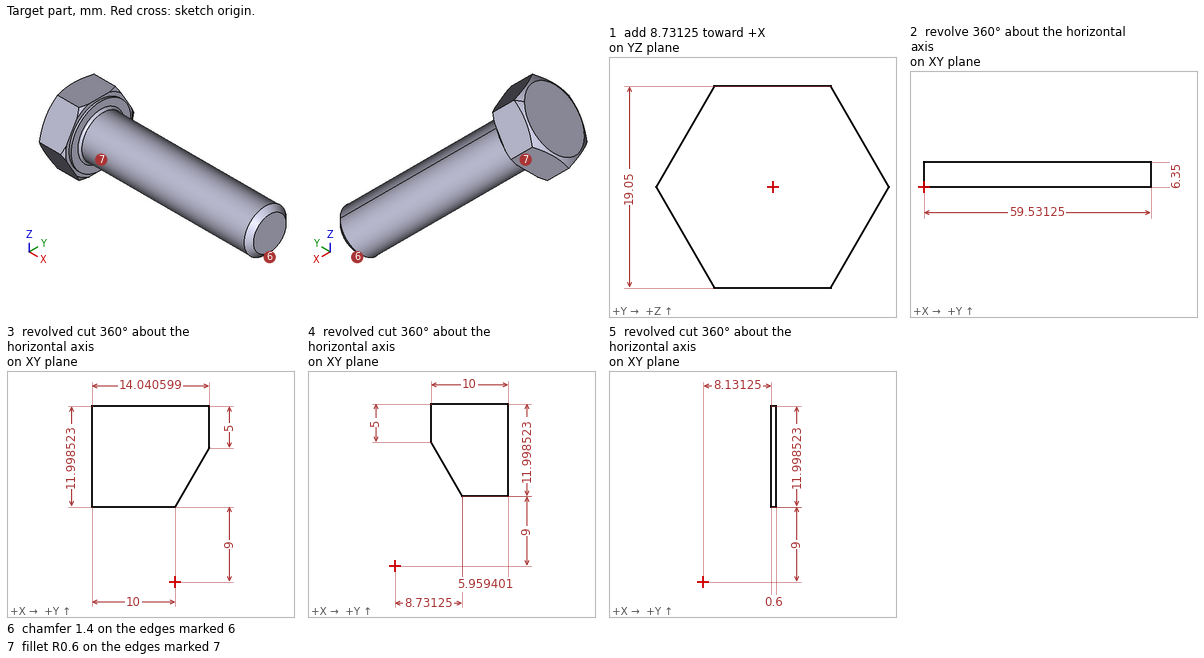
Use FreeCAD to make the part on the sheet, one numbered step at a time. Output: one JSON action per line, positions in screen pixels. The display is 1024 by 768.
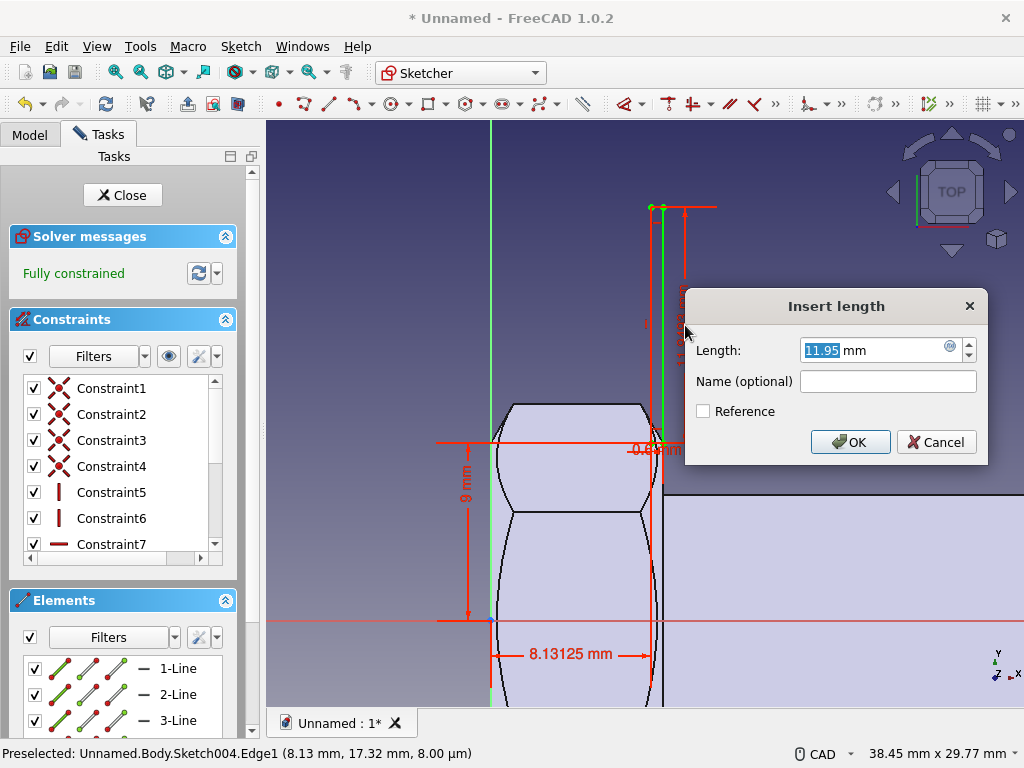
{"action": "type", "text": "11.998523"}
{"action": "key", "text": "Return"}
{"action": "key", "text": "Escape"}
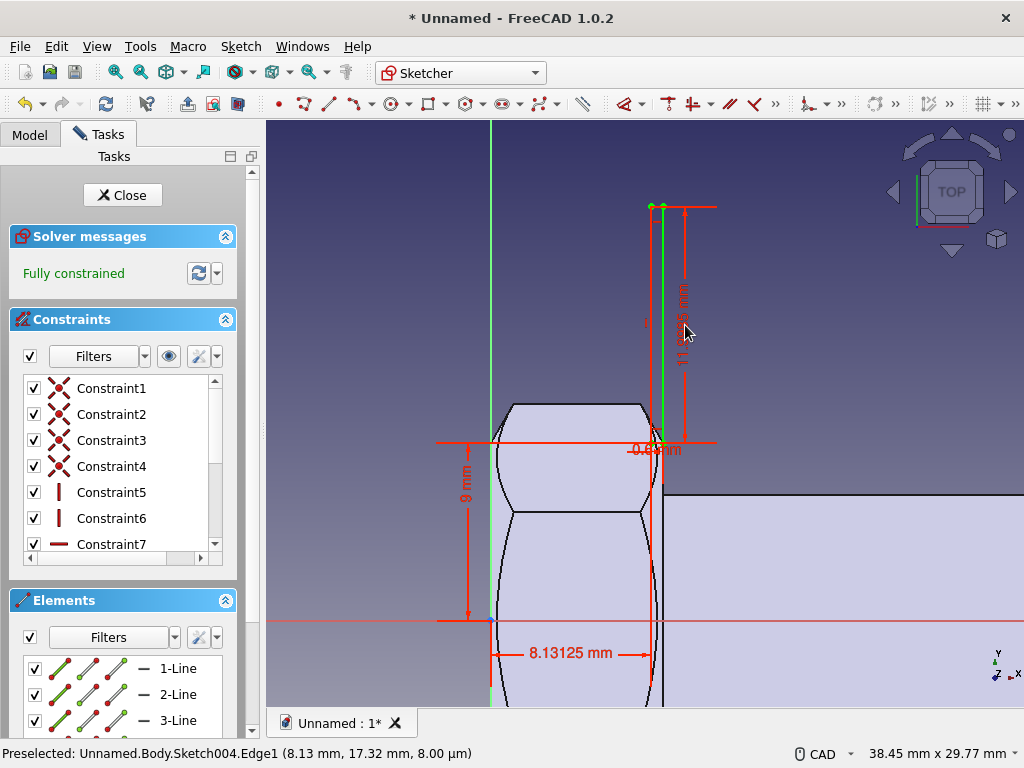
{"action": "left_click", "coordinate": [123, 195]}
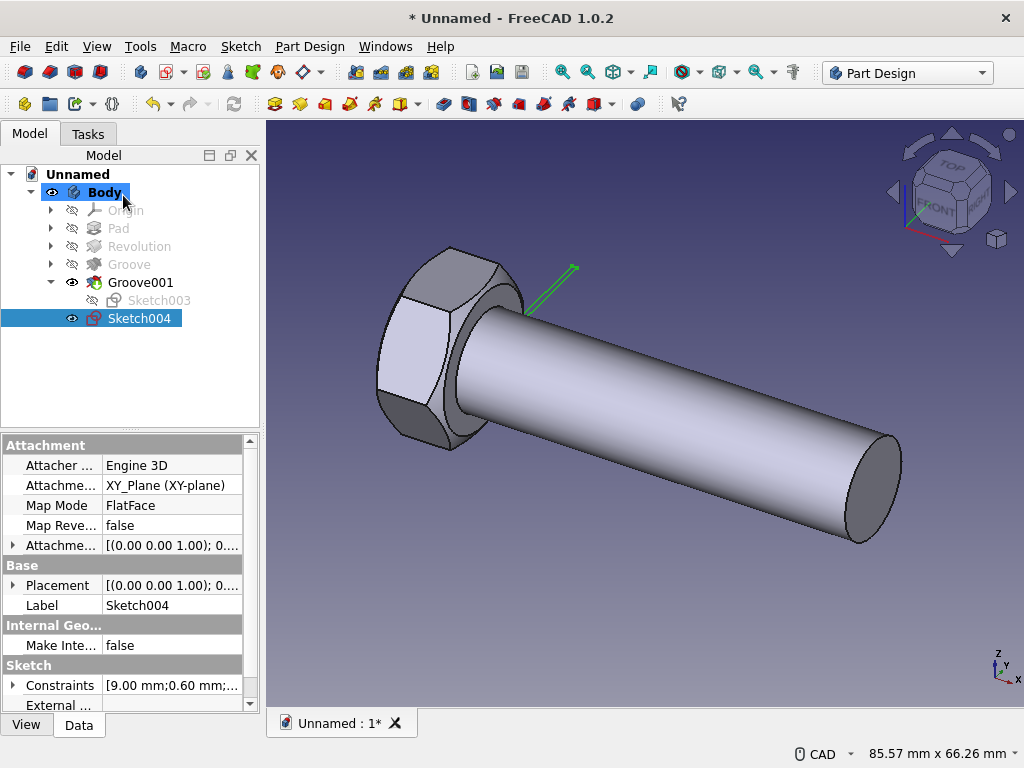
{"action": "left_click", "coordinate": [494, 104]}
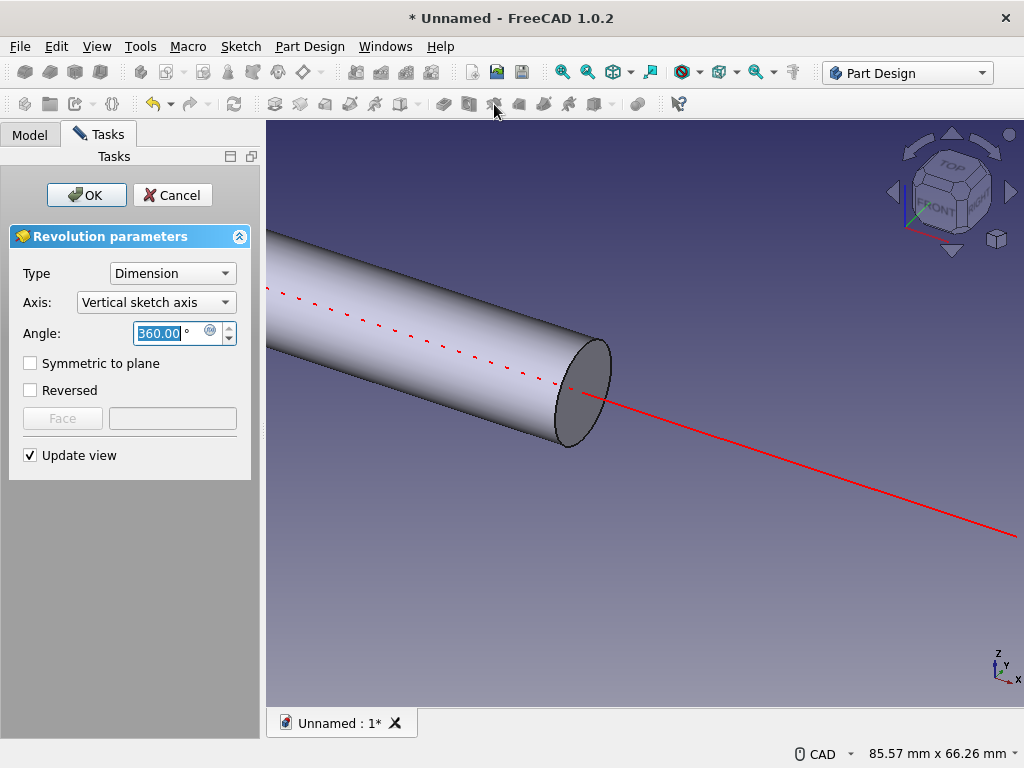
{"action": "left_click", "coordinate": [157, 302]}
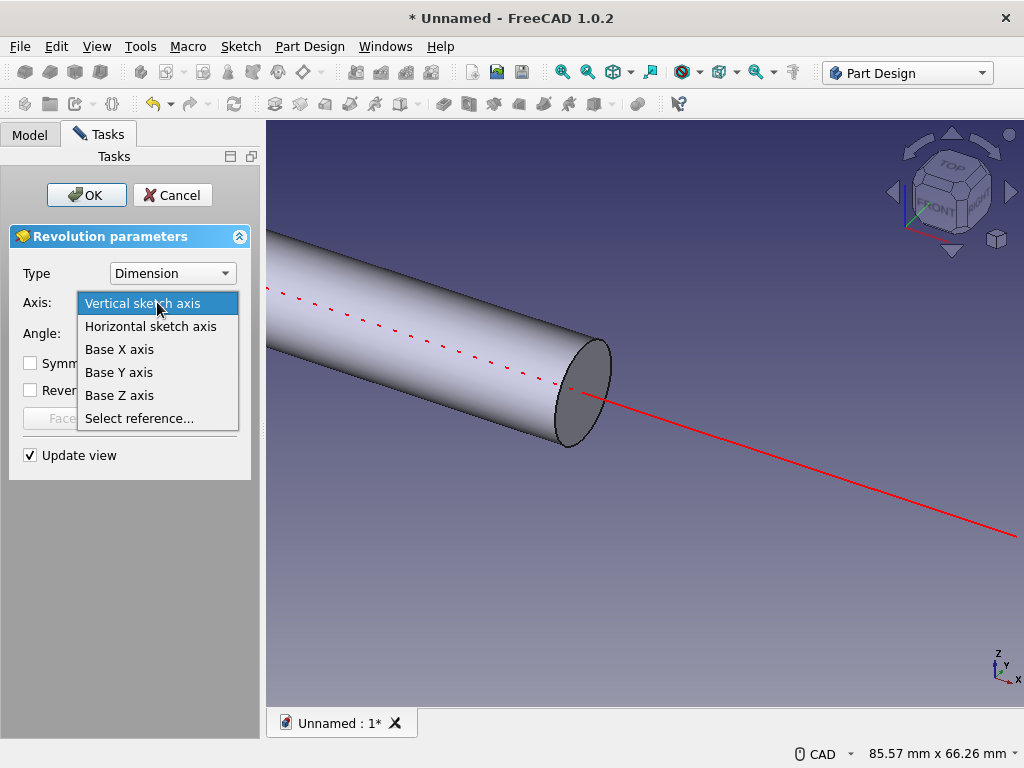
{"action": "left_click", "coordinate": [156, 326]}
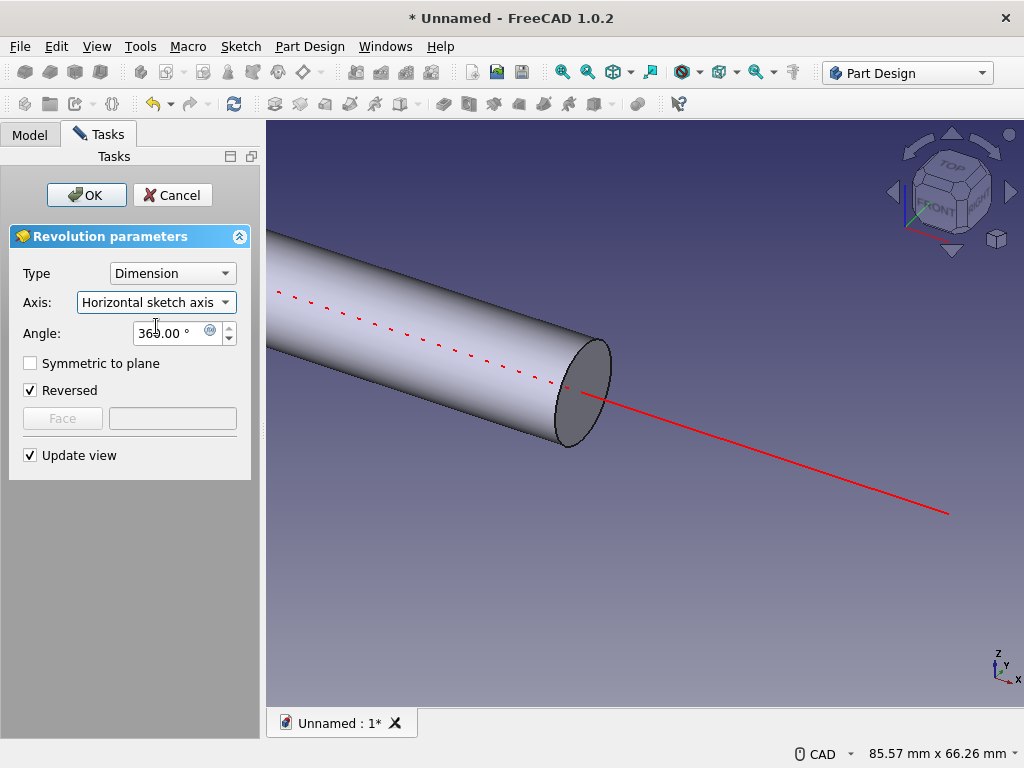
{"action": "left_click", "coordinate": [87, 195]}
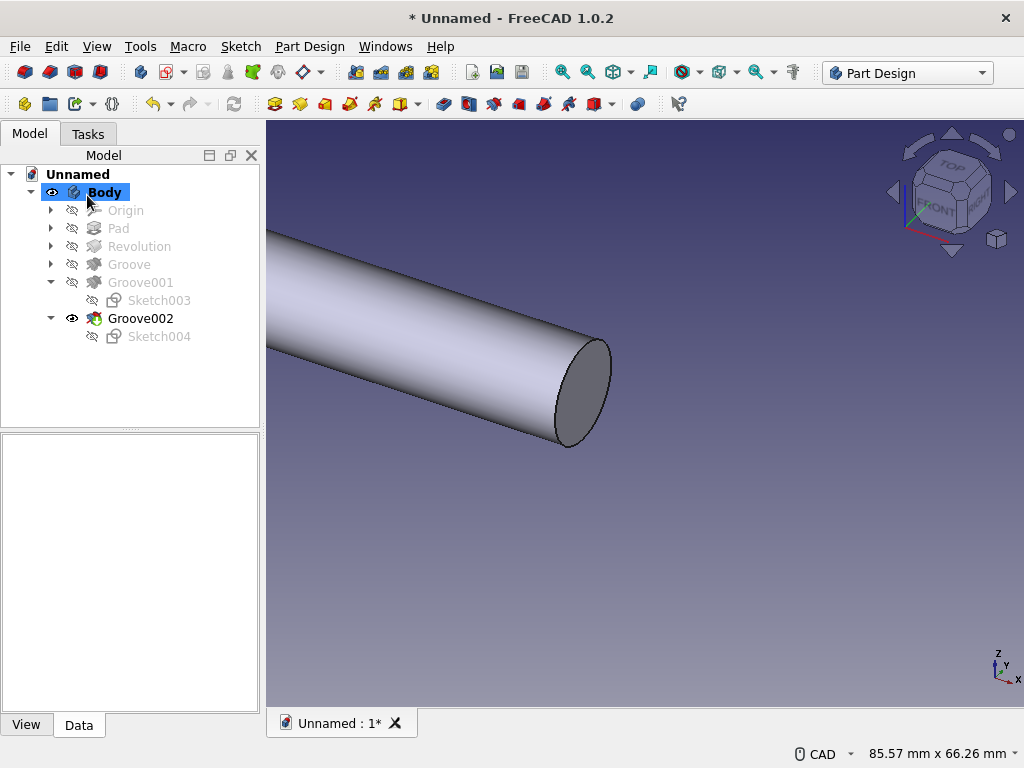
{"action": "left_click", "coordinate": [563, 72]}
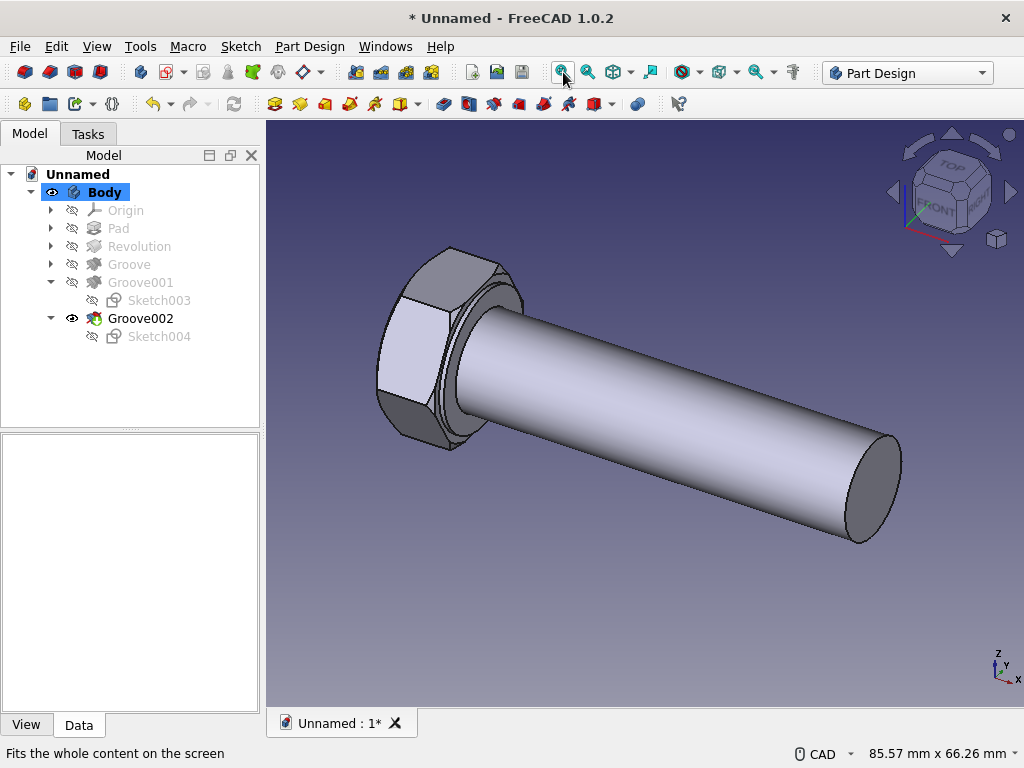
{"action": "left_click", "coordinate": [845, 516]}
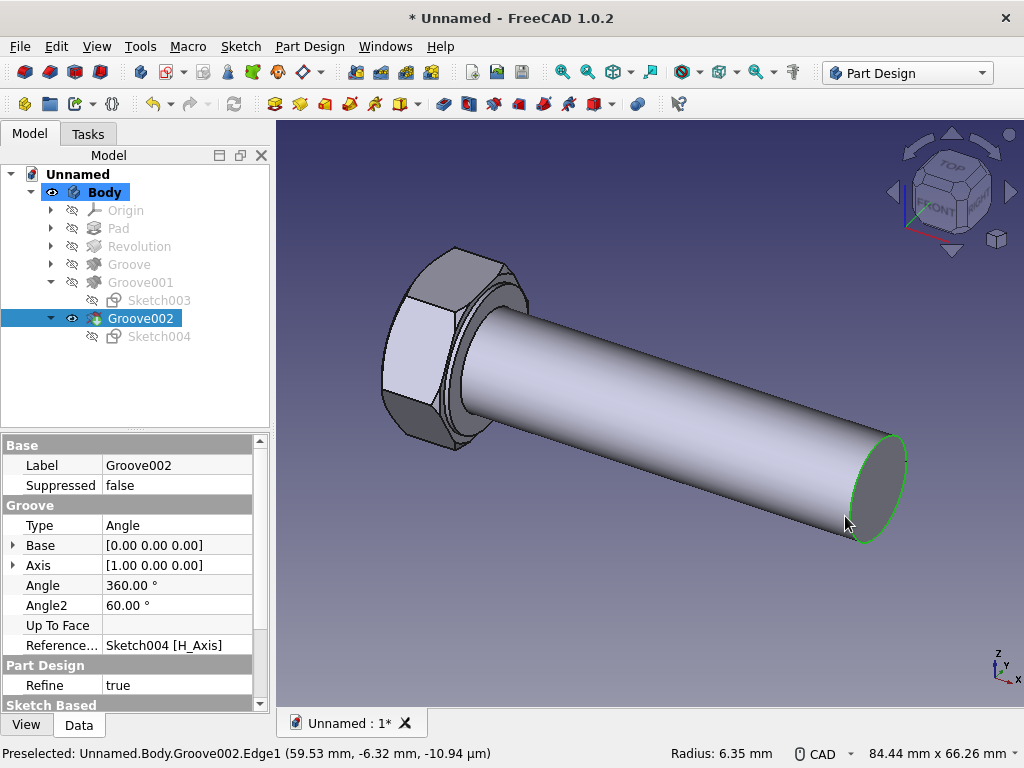
{"action": "left_click", "coordinate": [50, 72]}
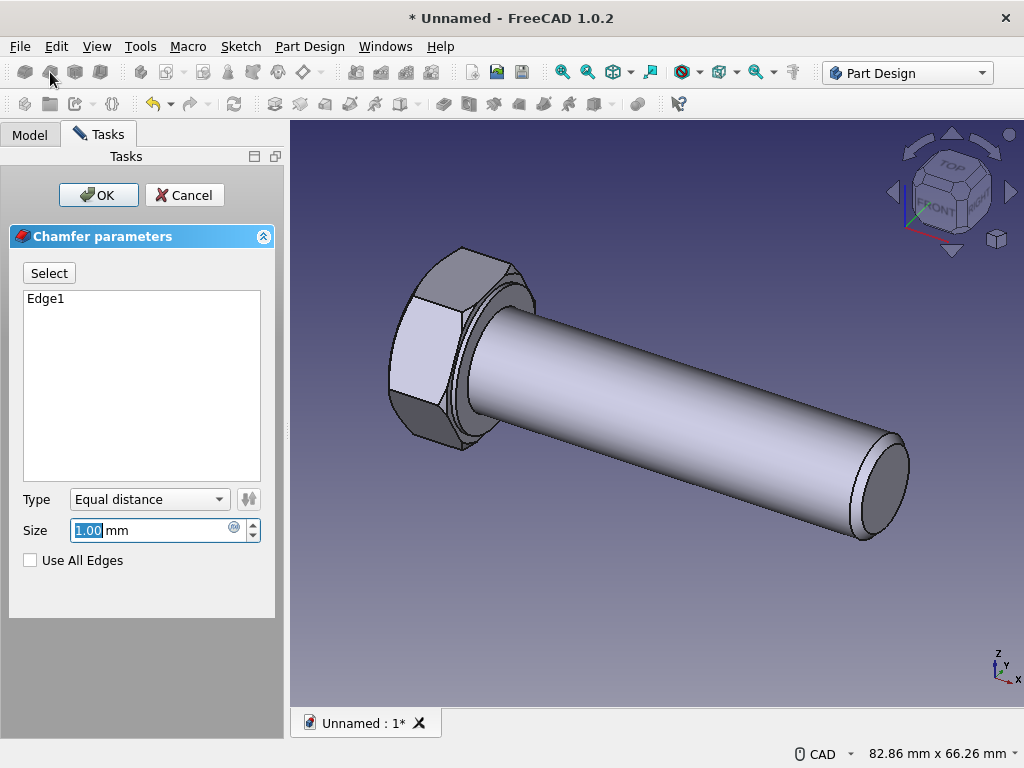
{"action": "type", "text": "1.4"}
{"action": "key", "text": "Tab"}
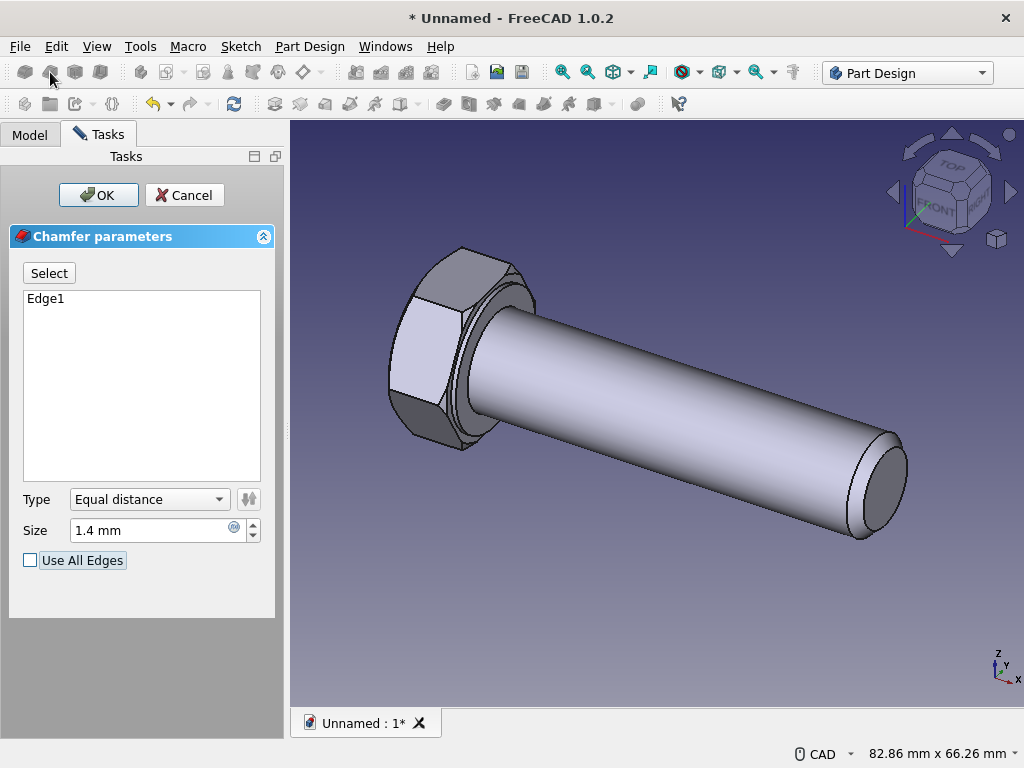
{"action": "left_click", "coordinate": [99, 195]}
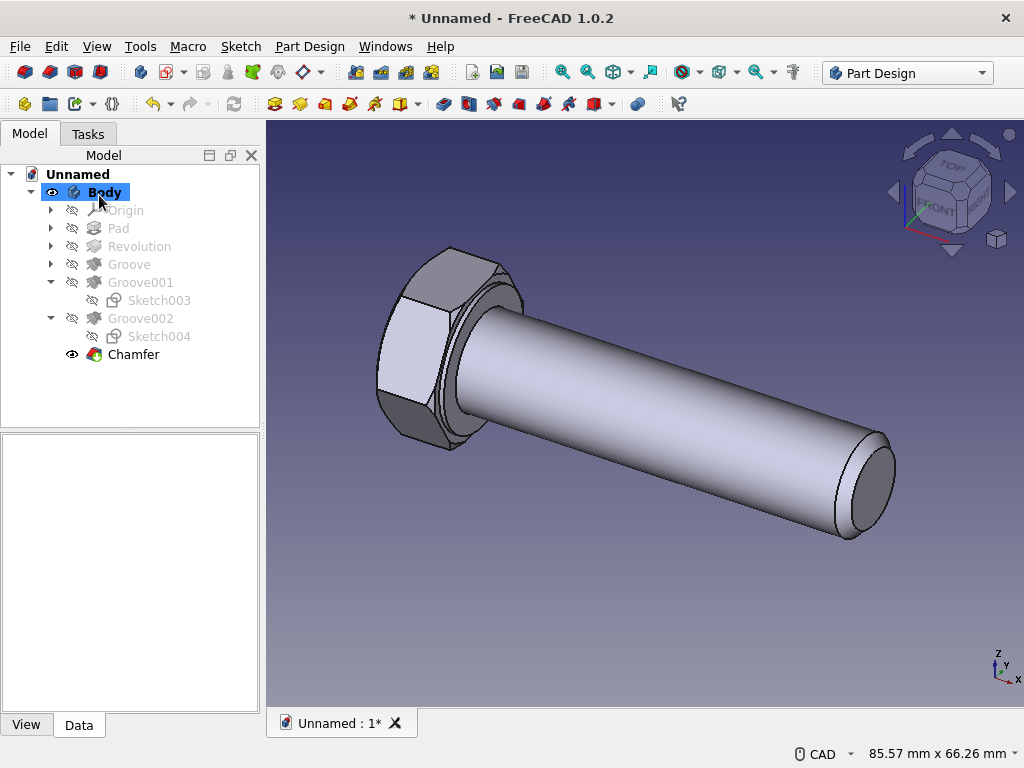
{"action": "key", "text": "0"}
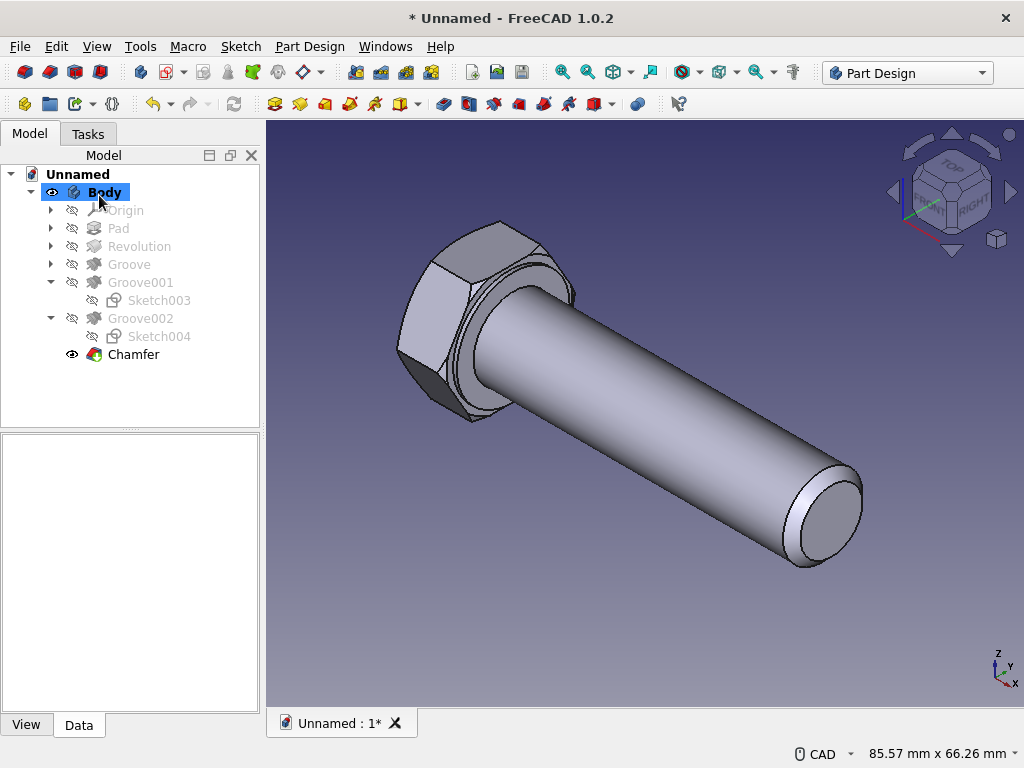
{"action": "key", "text": "2"}